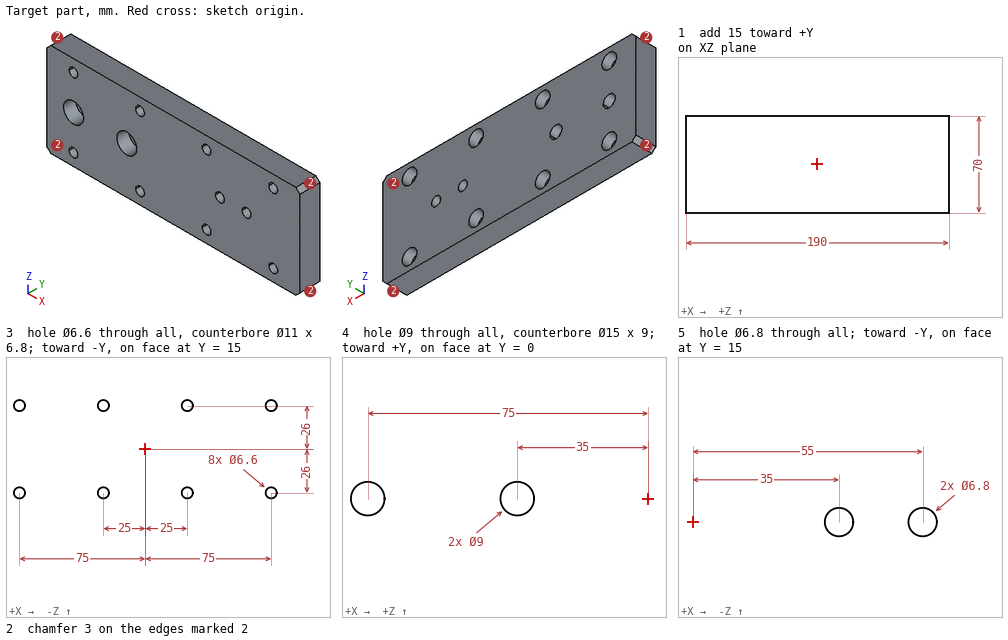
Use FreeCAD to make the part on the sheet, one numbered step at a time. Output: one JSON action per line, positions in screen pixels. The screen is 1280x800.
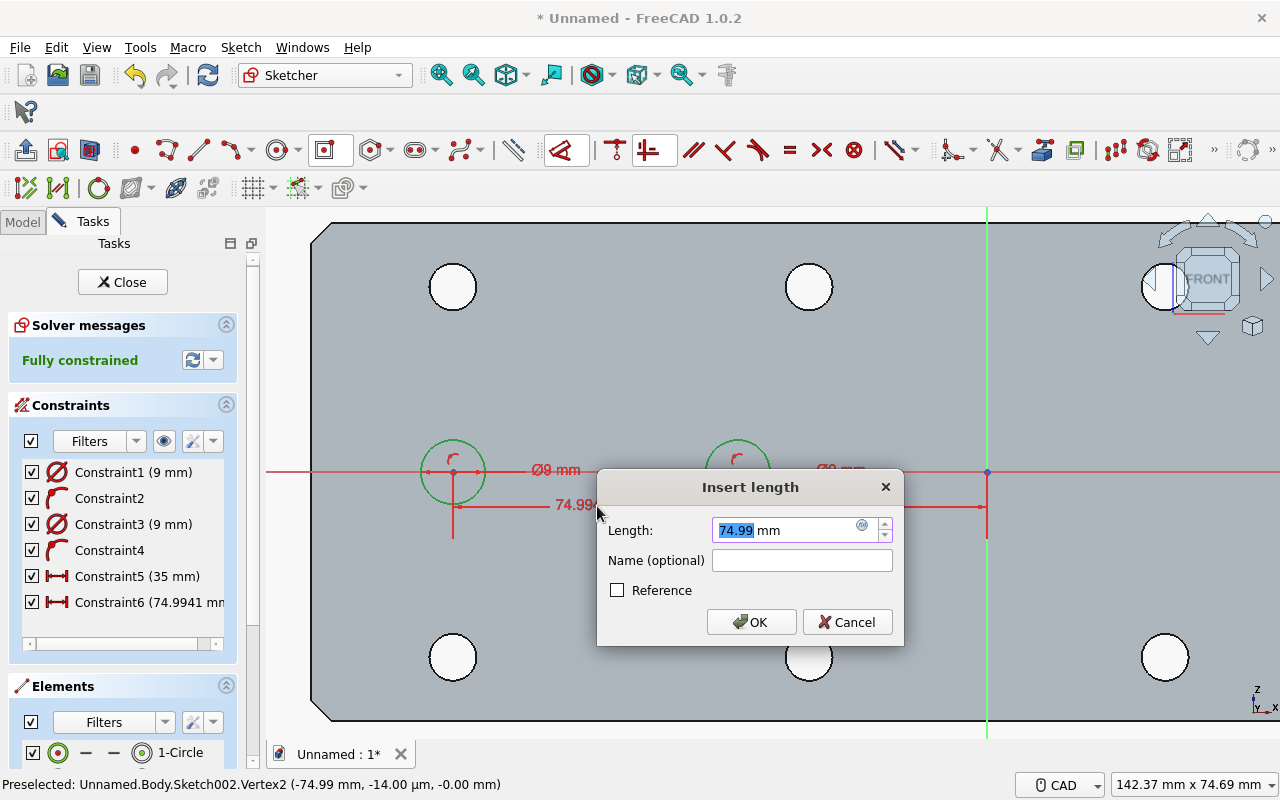
{"action": "type", "text": "75"}
{"action": "key", "text": "Return"}
{"action": "key", "text": "Escape"}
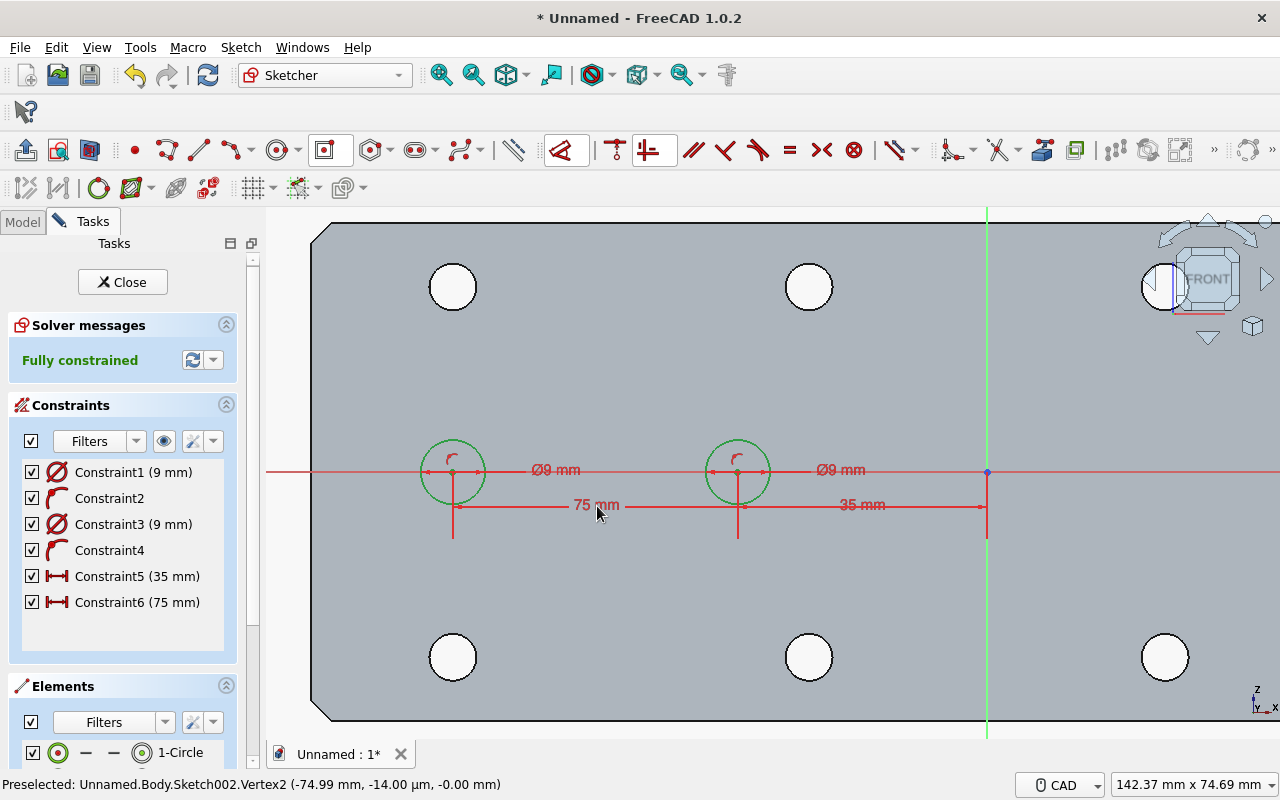
{"action": "left_click", "coordinate": [123, 282]}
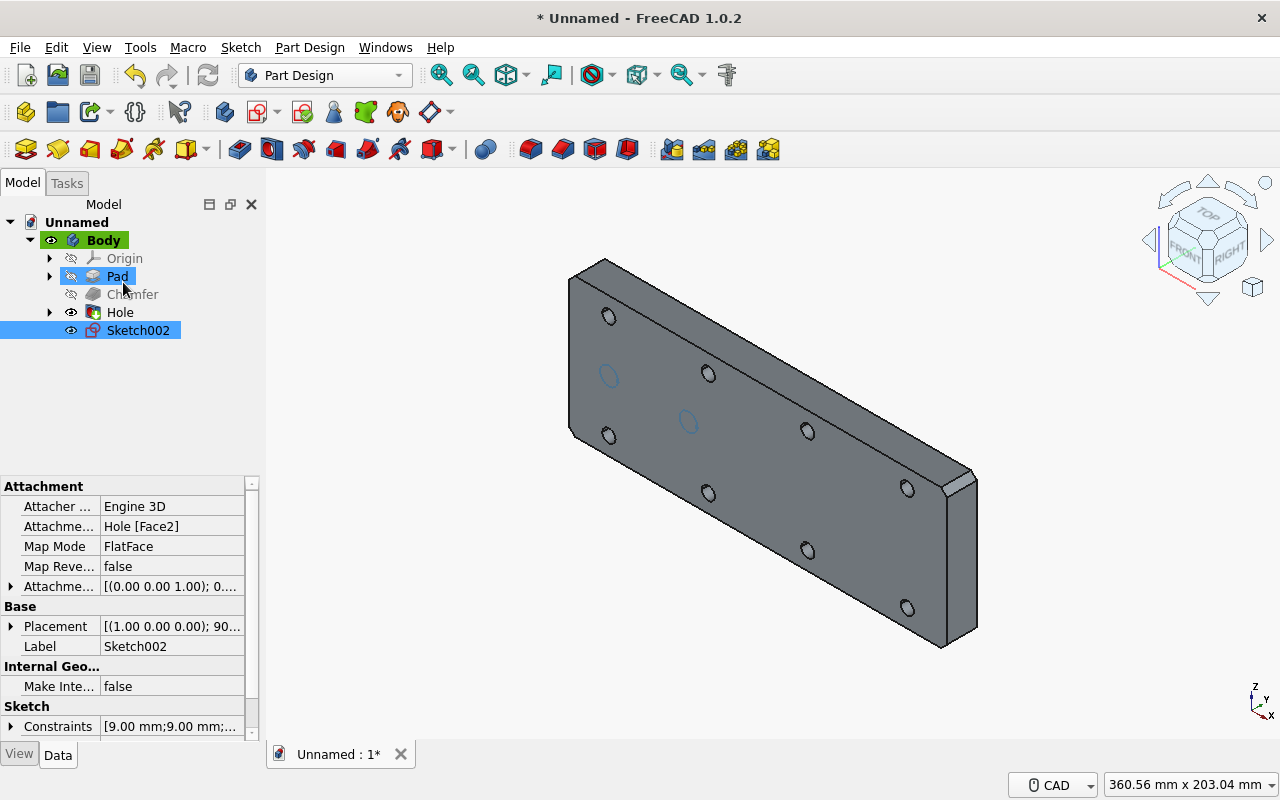
{"action": "left_click", "coordinate": [272, 150]}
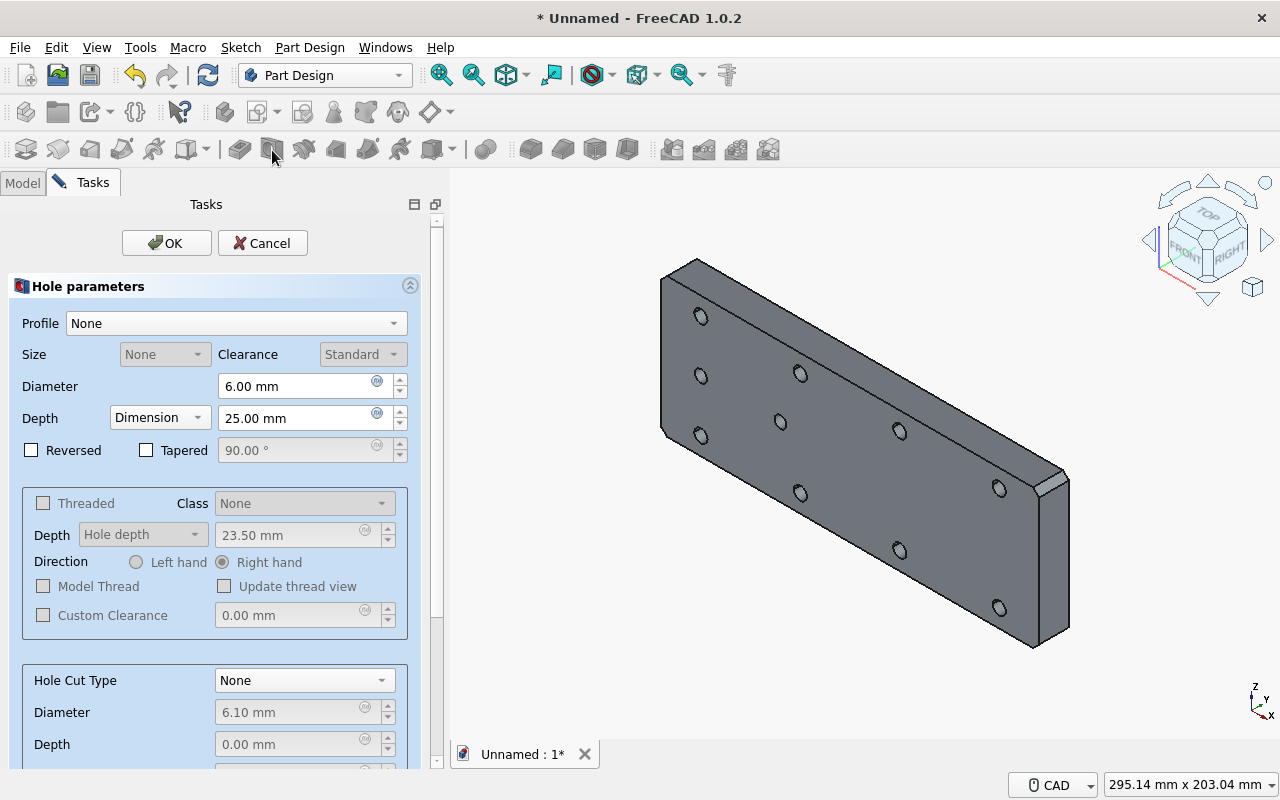
{"action": "triple_click", "coordinate": [305, 386]}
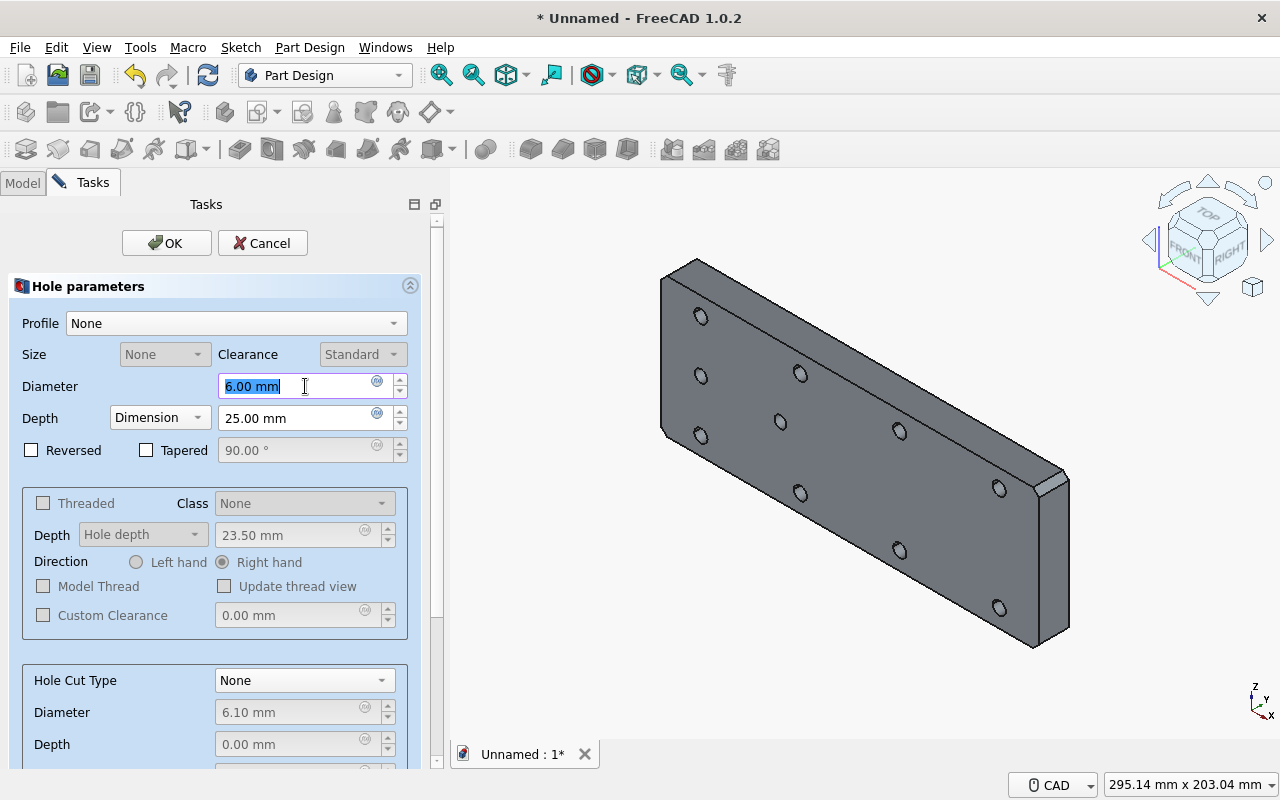
{"action": "type", "text": "9"}
{"action": "key", "text": "Tab"}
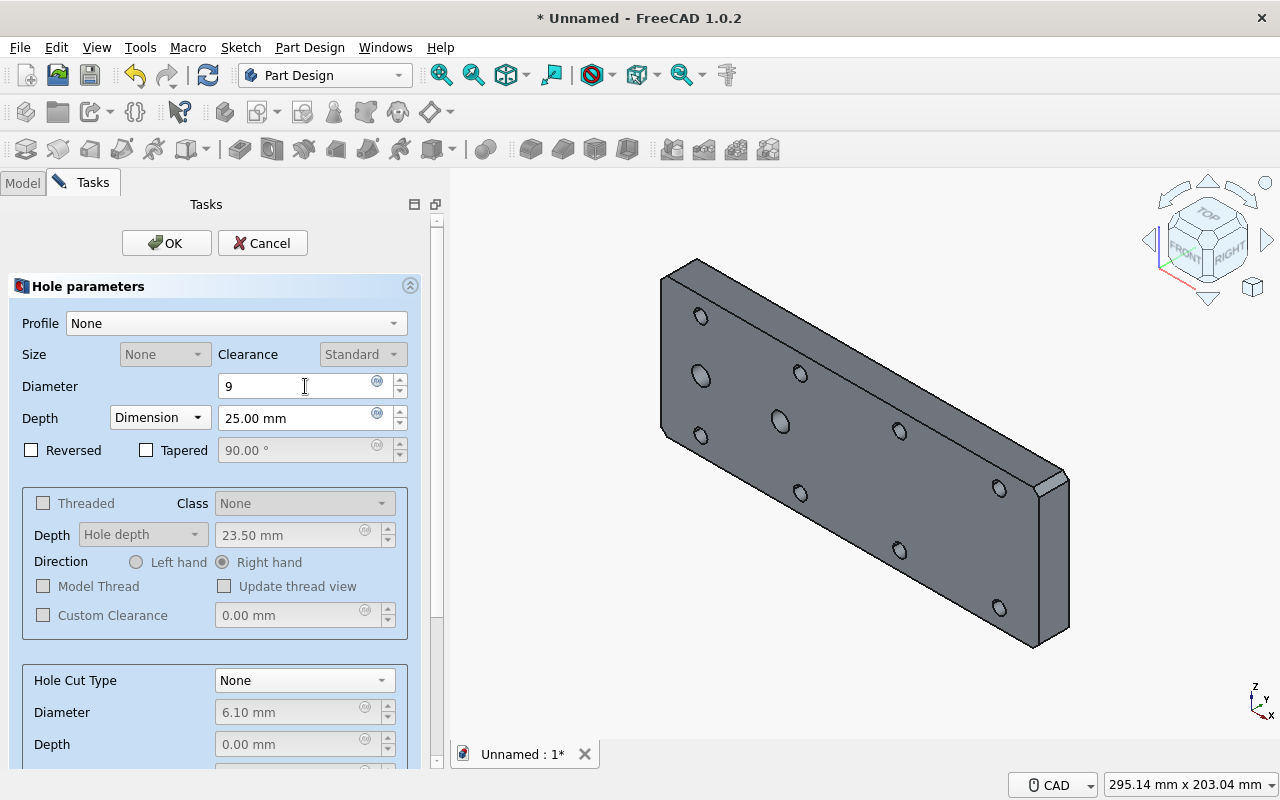
{"action": "left_click", "coordinate": [161, 418]}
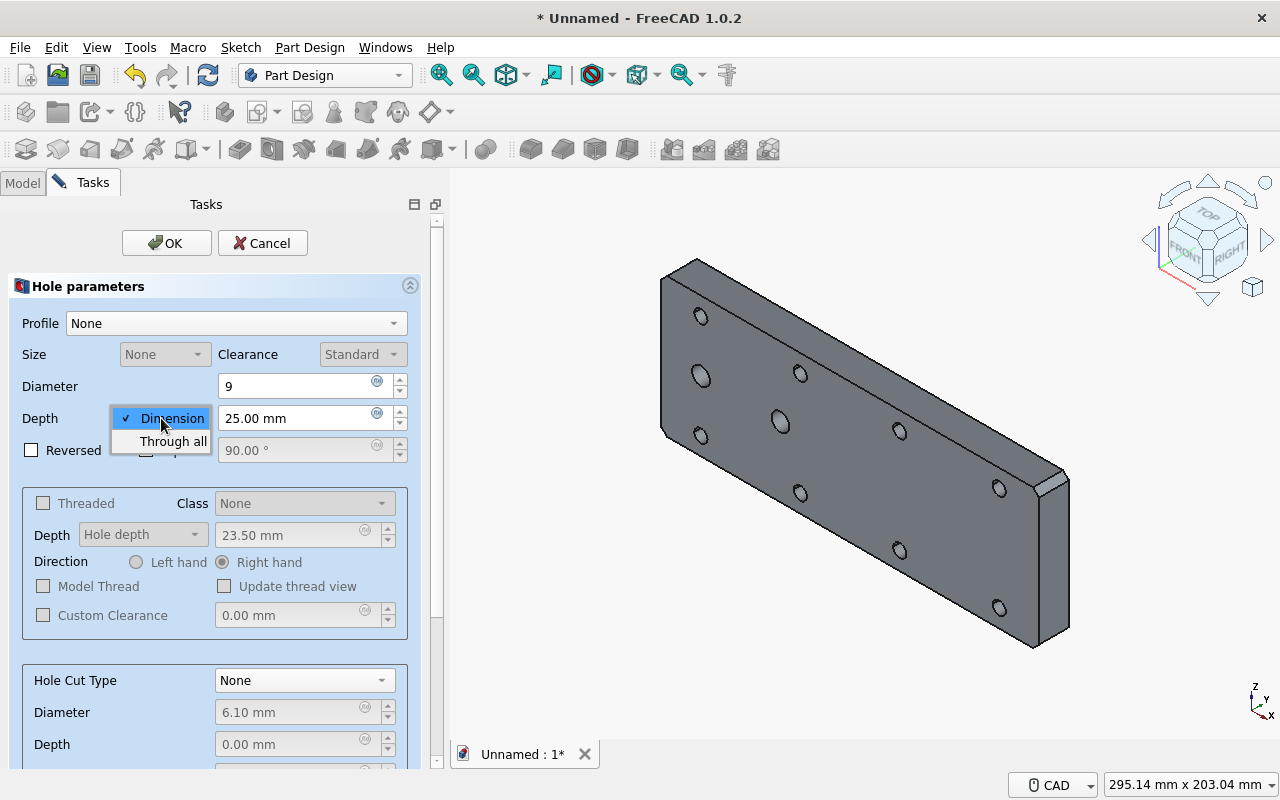
{"action": "left_click", "coordinate": [160, 442]}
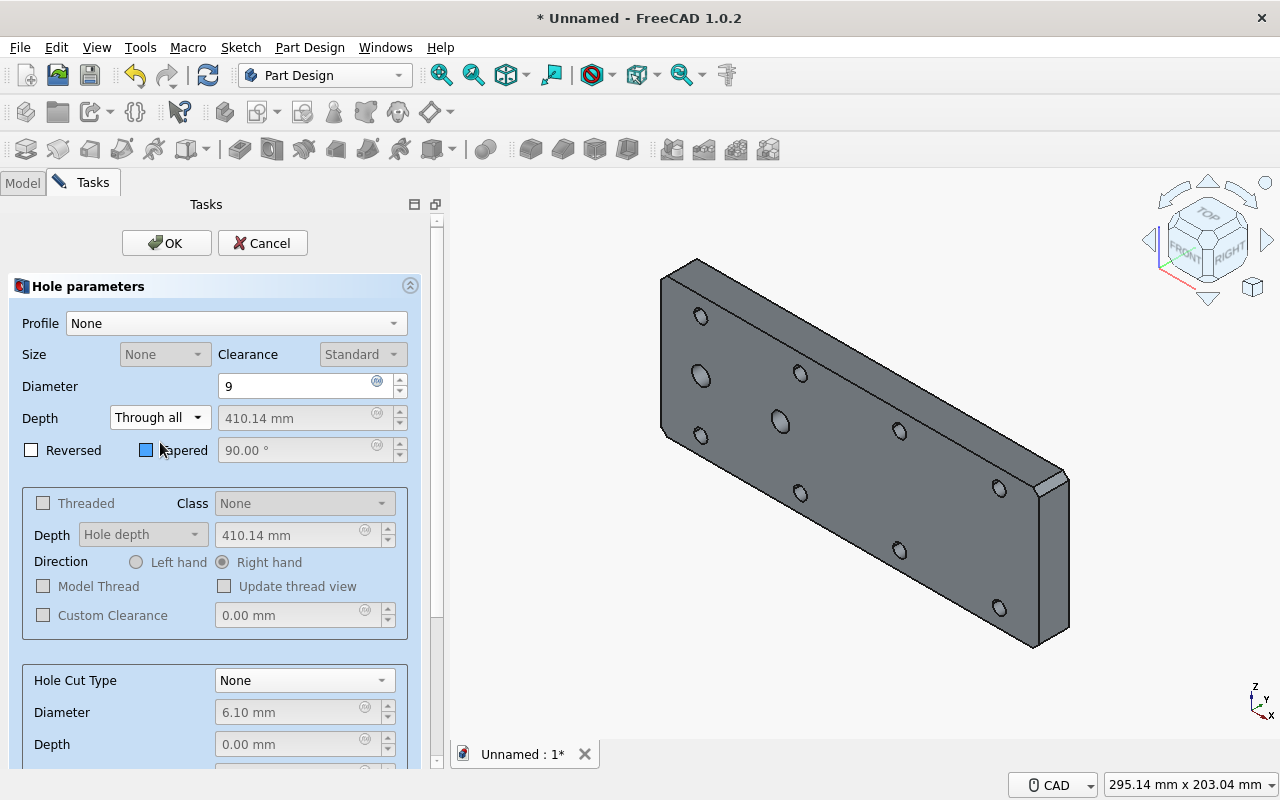
{"action": "left_click", "coordinate": [306, 680]}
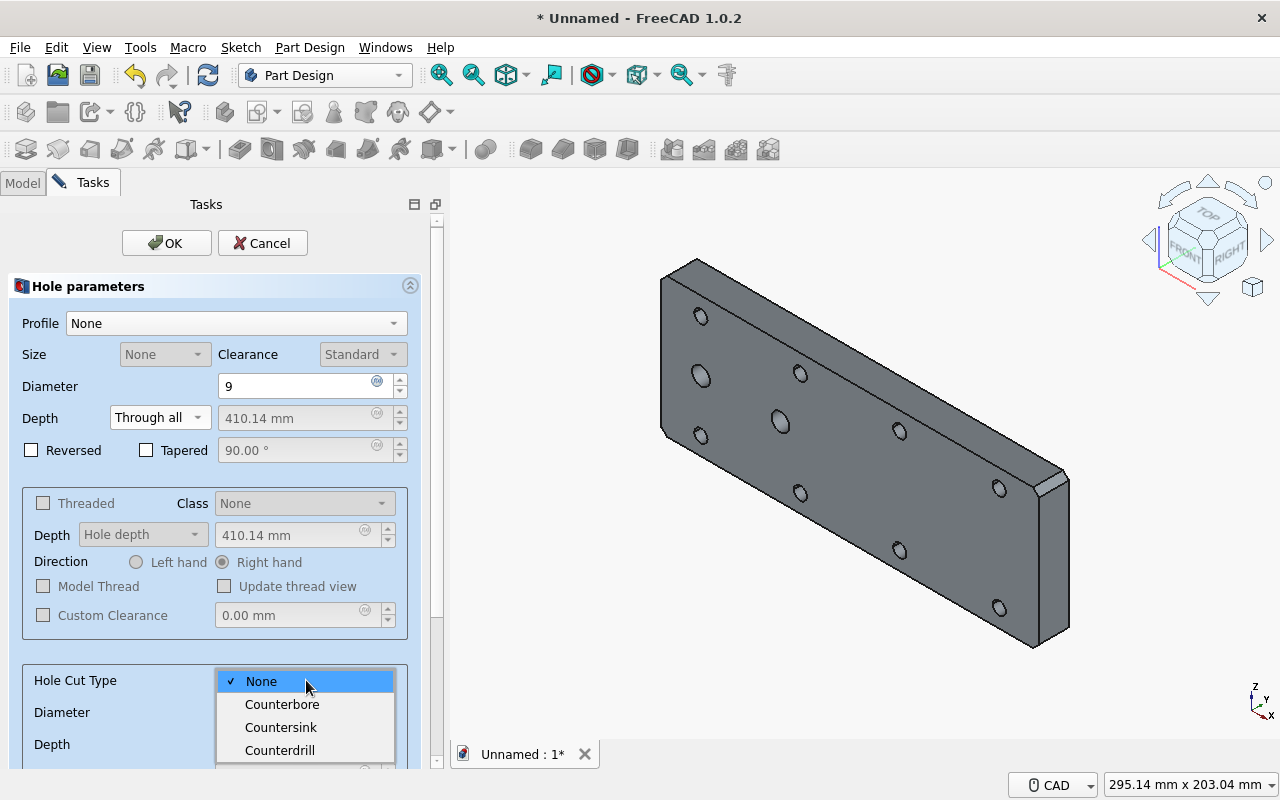
{"action": "left_click", "coordinate": [304, 704]}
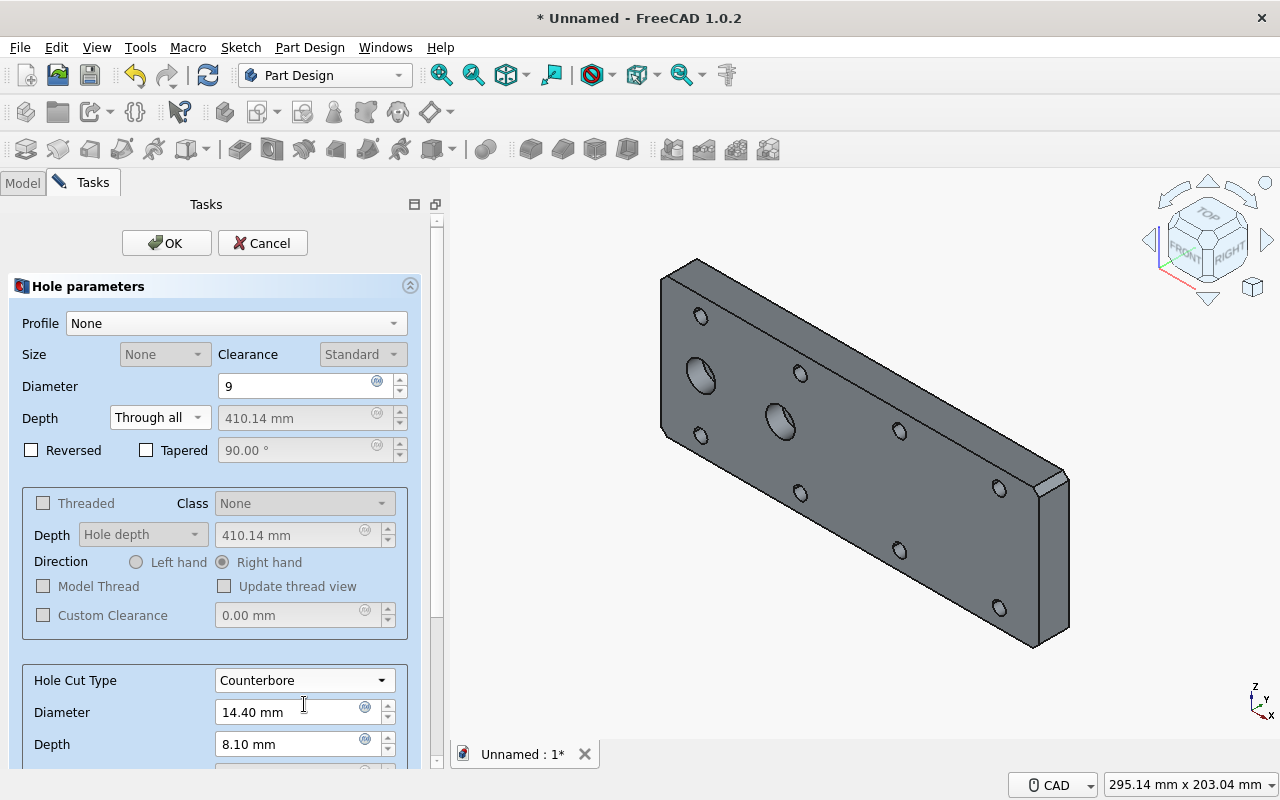
{"action": "triple_click", "coordinate": [298, 712]}